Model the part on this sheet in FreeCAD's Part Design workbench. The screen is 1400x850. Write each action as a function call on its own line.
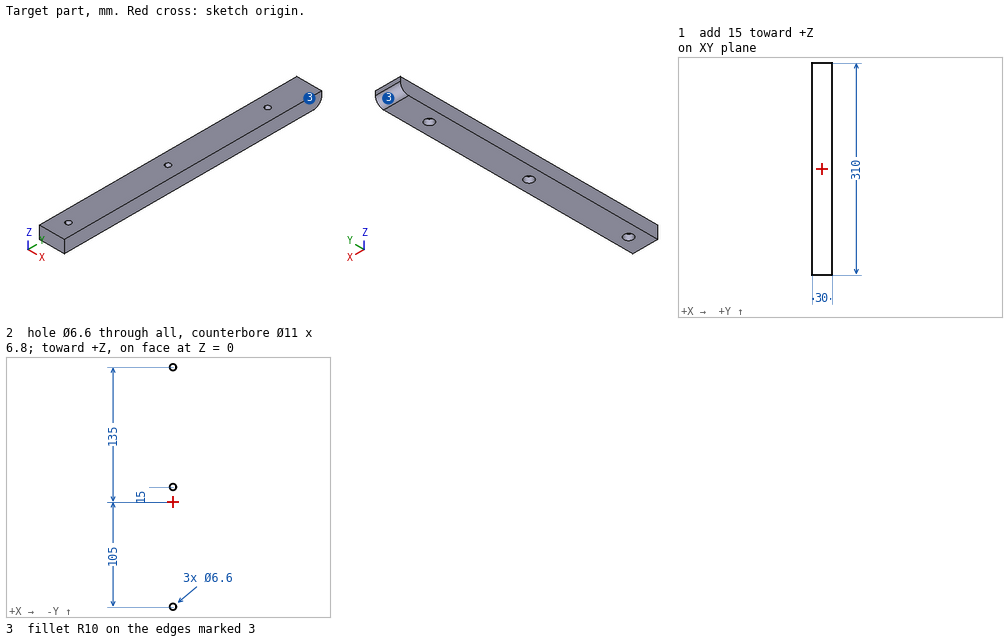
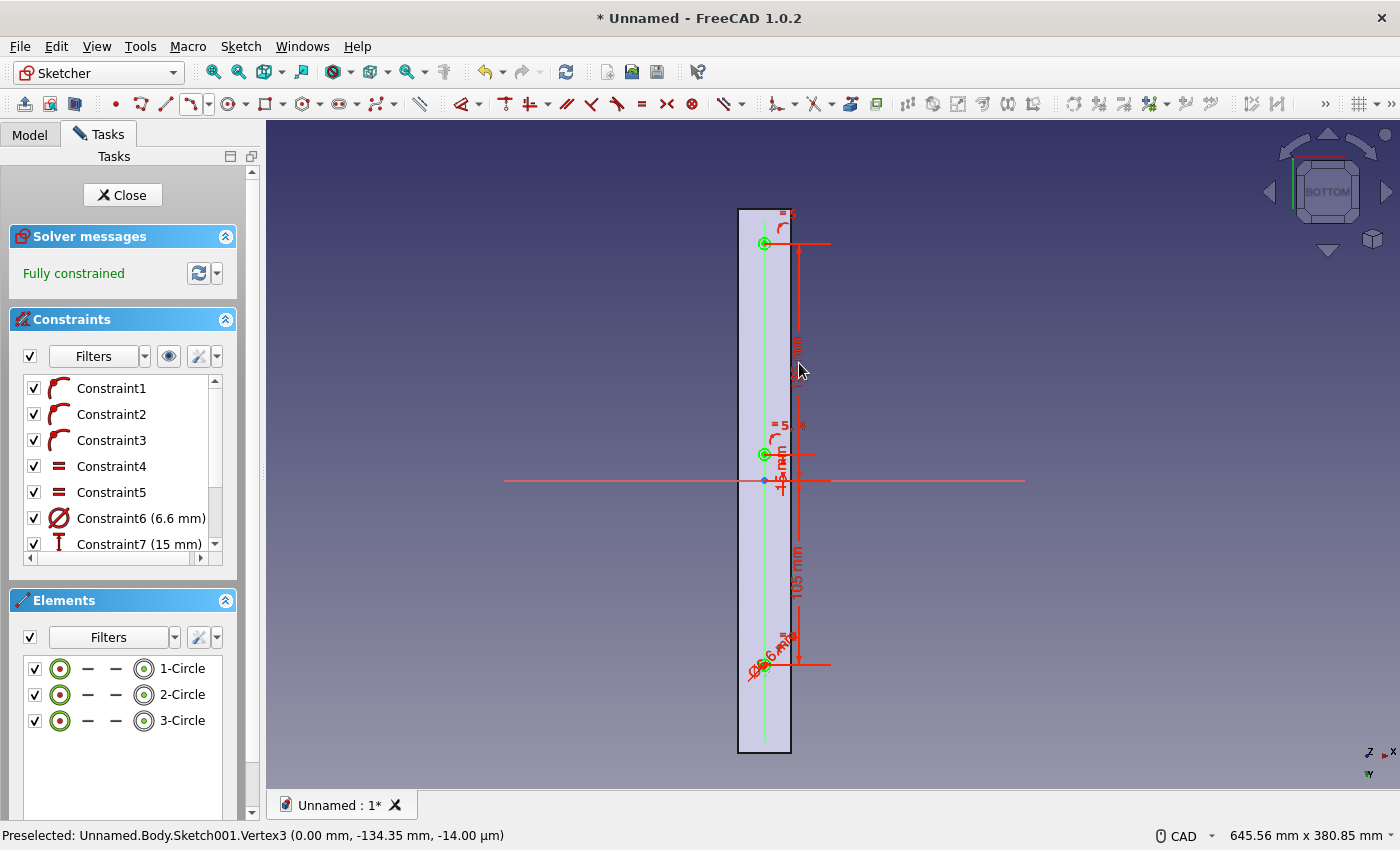
click(123, 195)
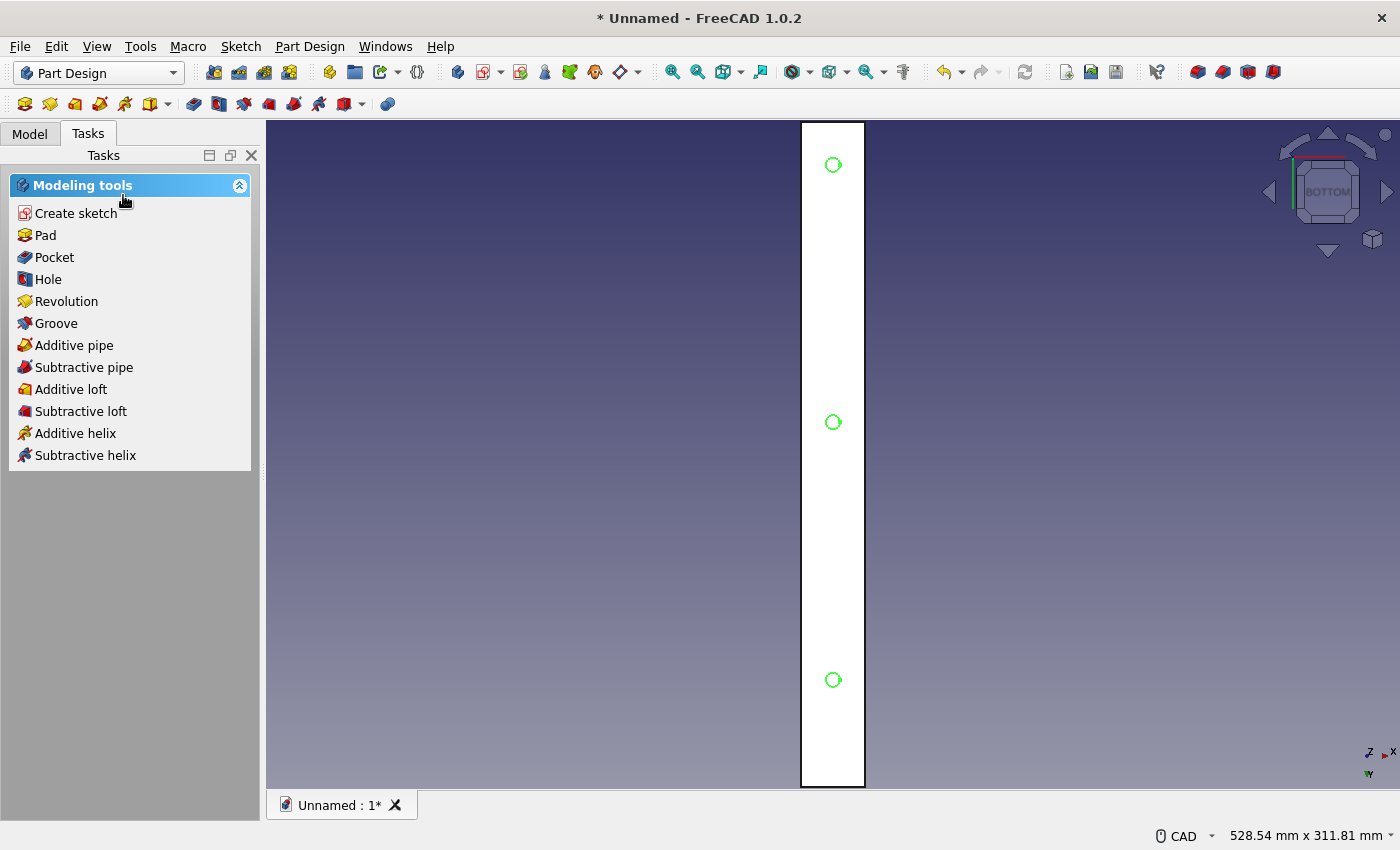
click(219, 104)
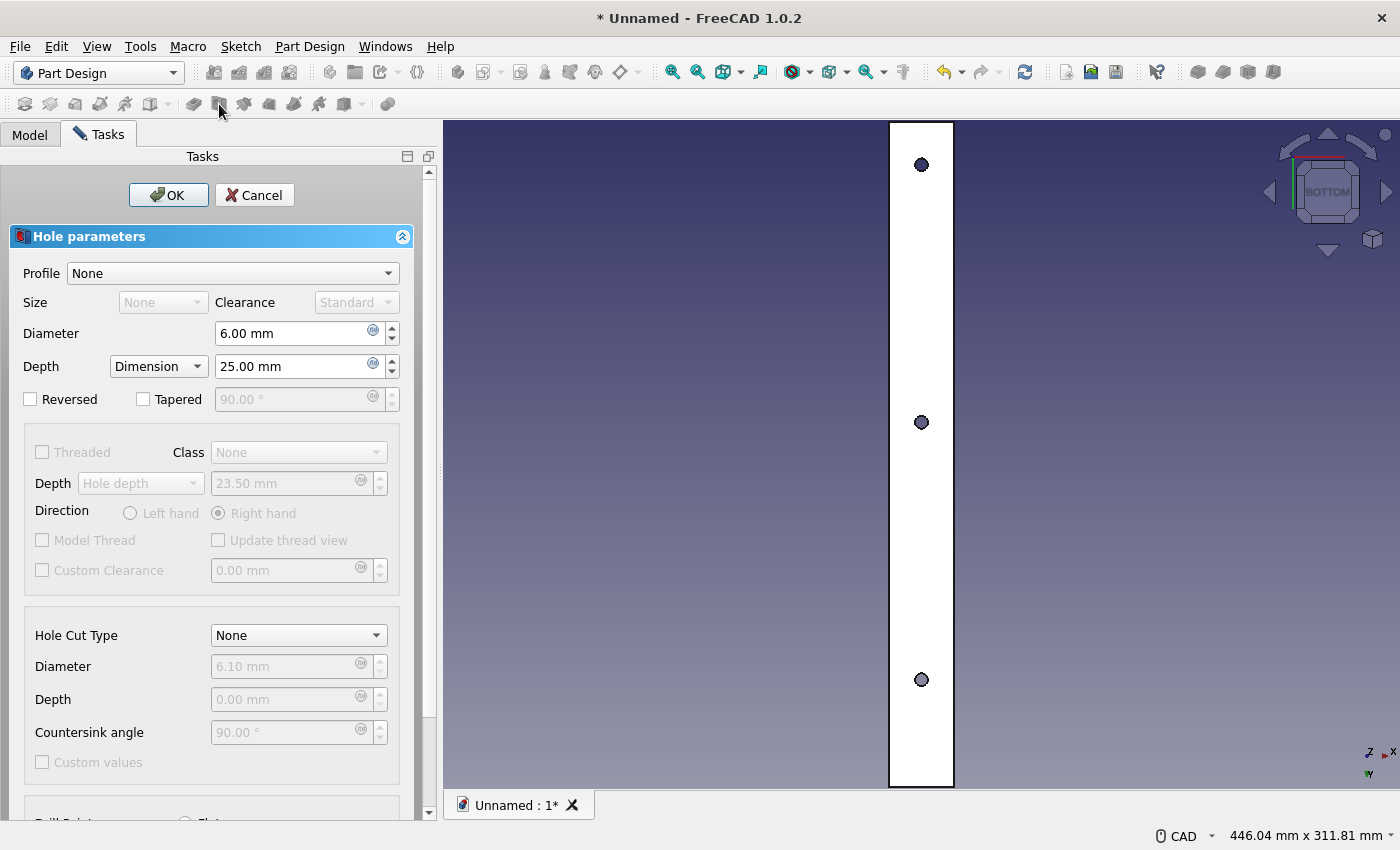
triple_click(300, 334)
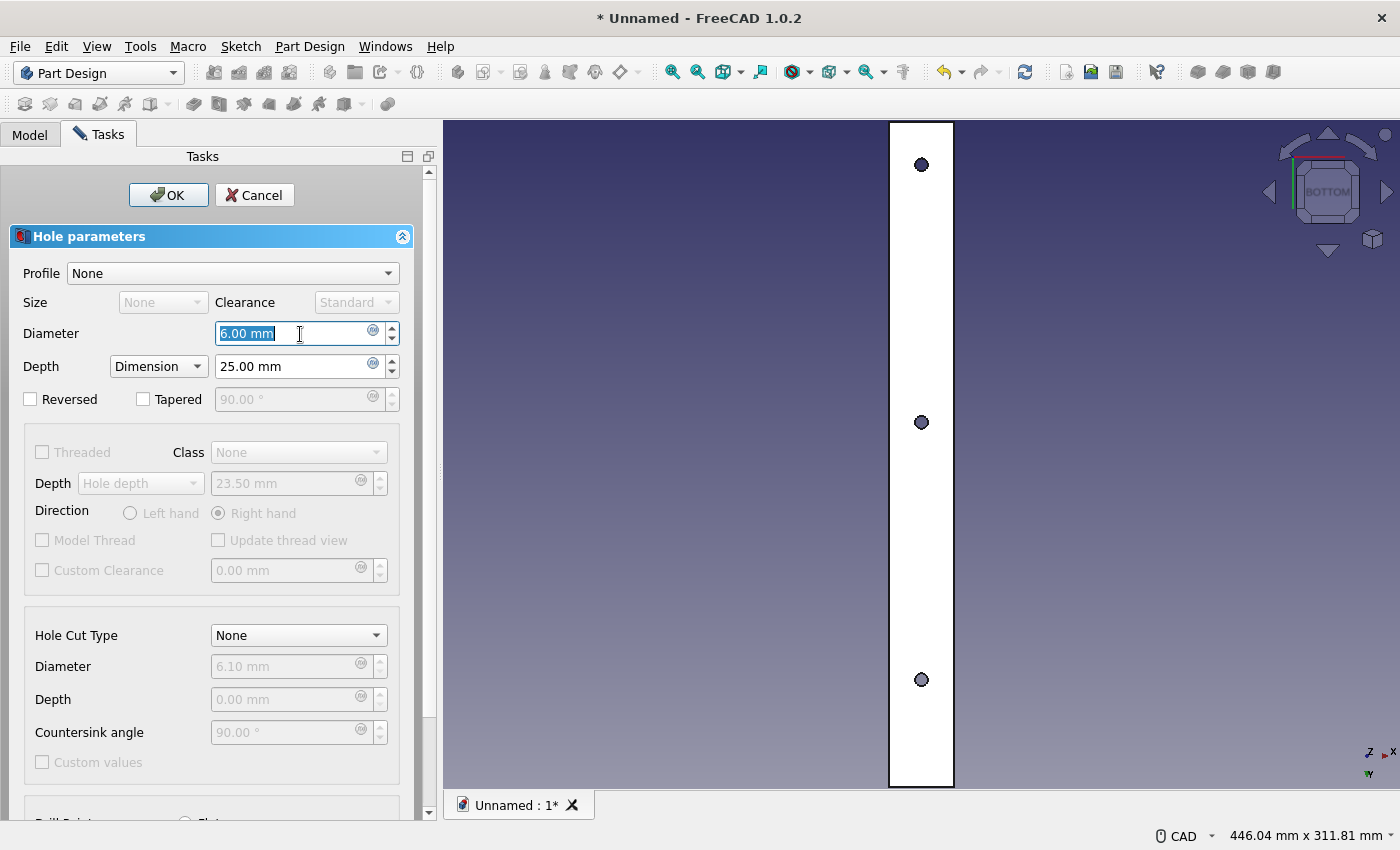
text(6.6)
key(Tab)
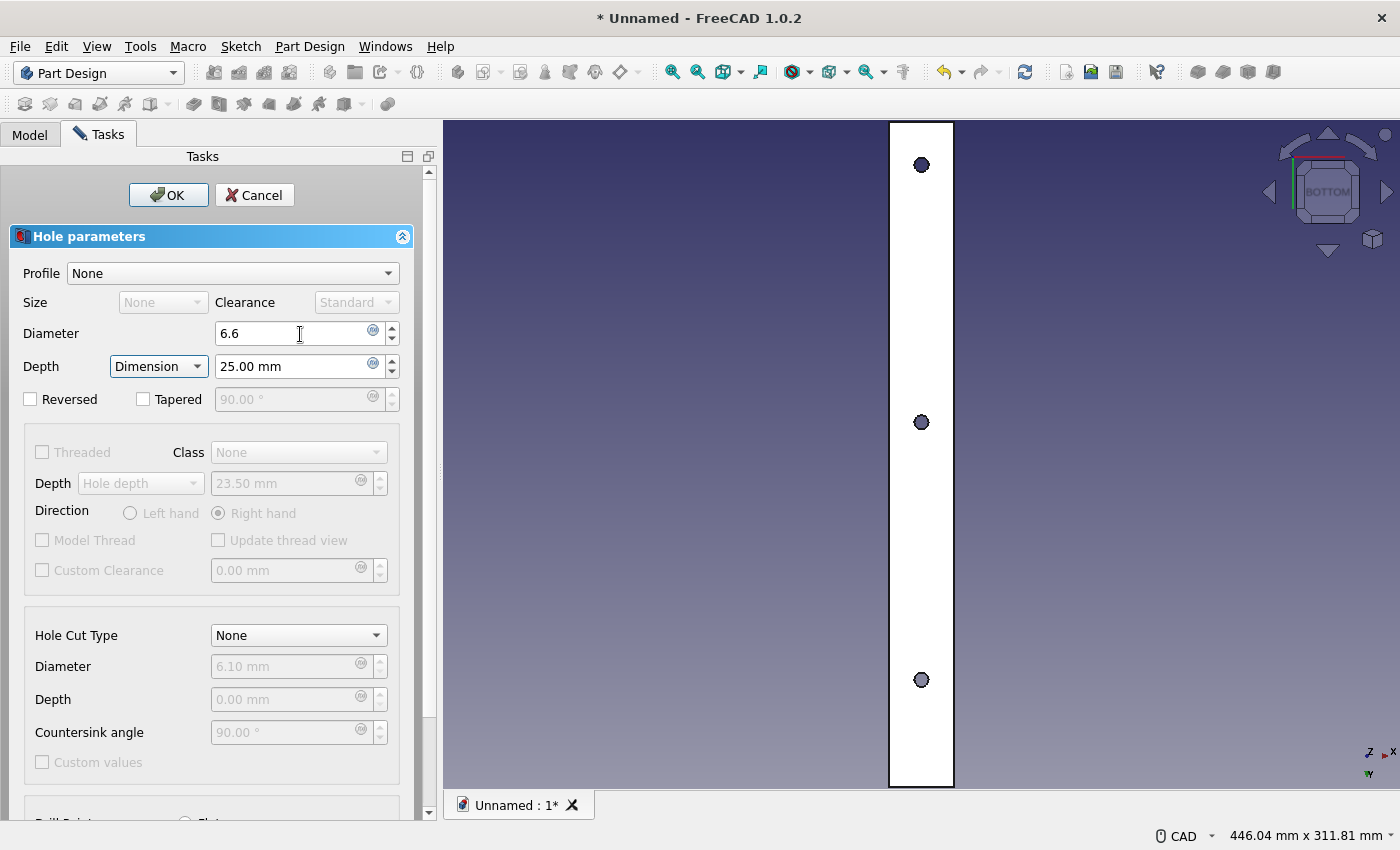
click(160, 366)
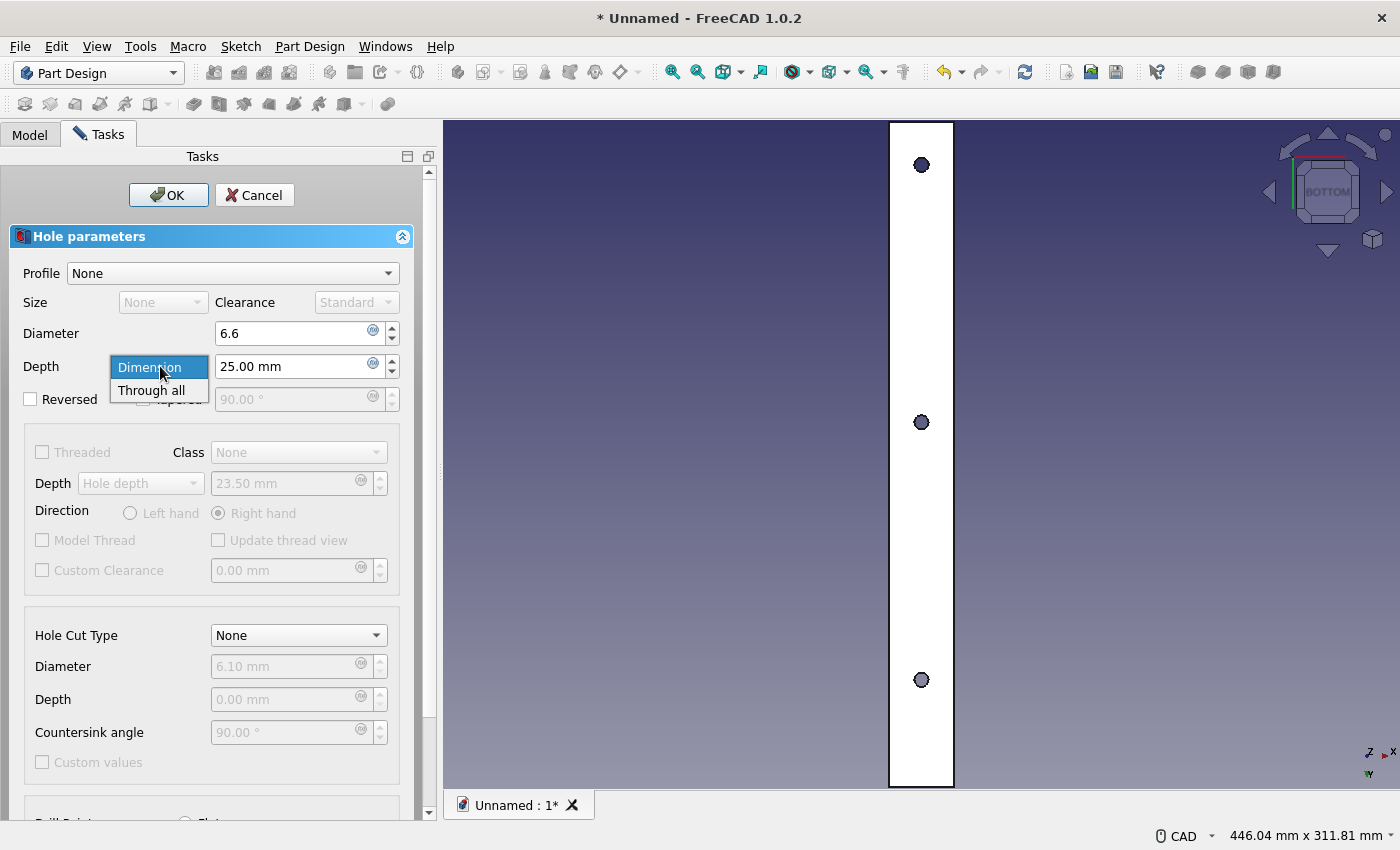
click(158, 390)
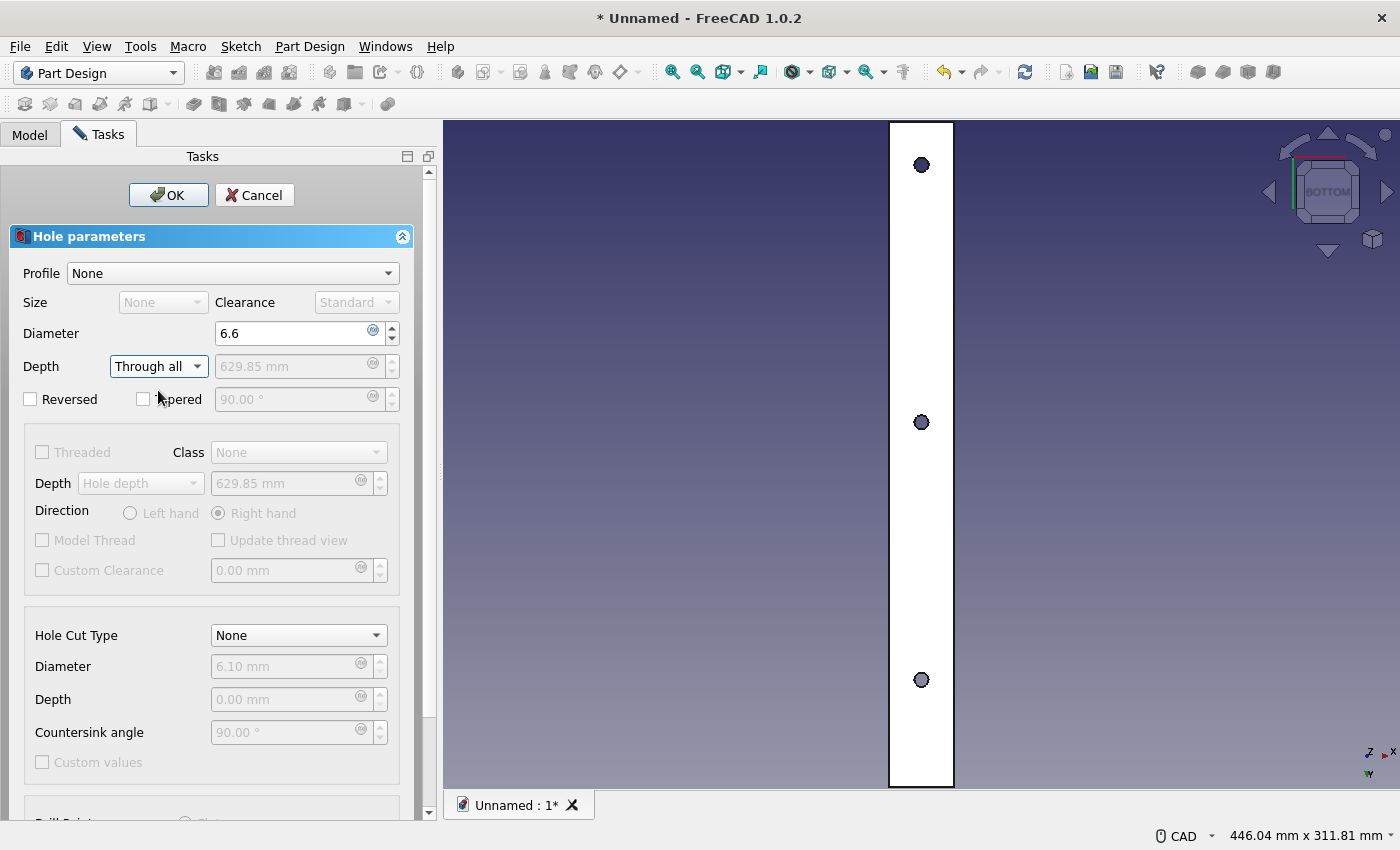
click(300, 636)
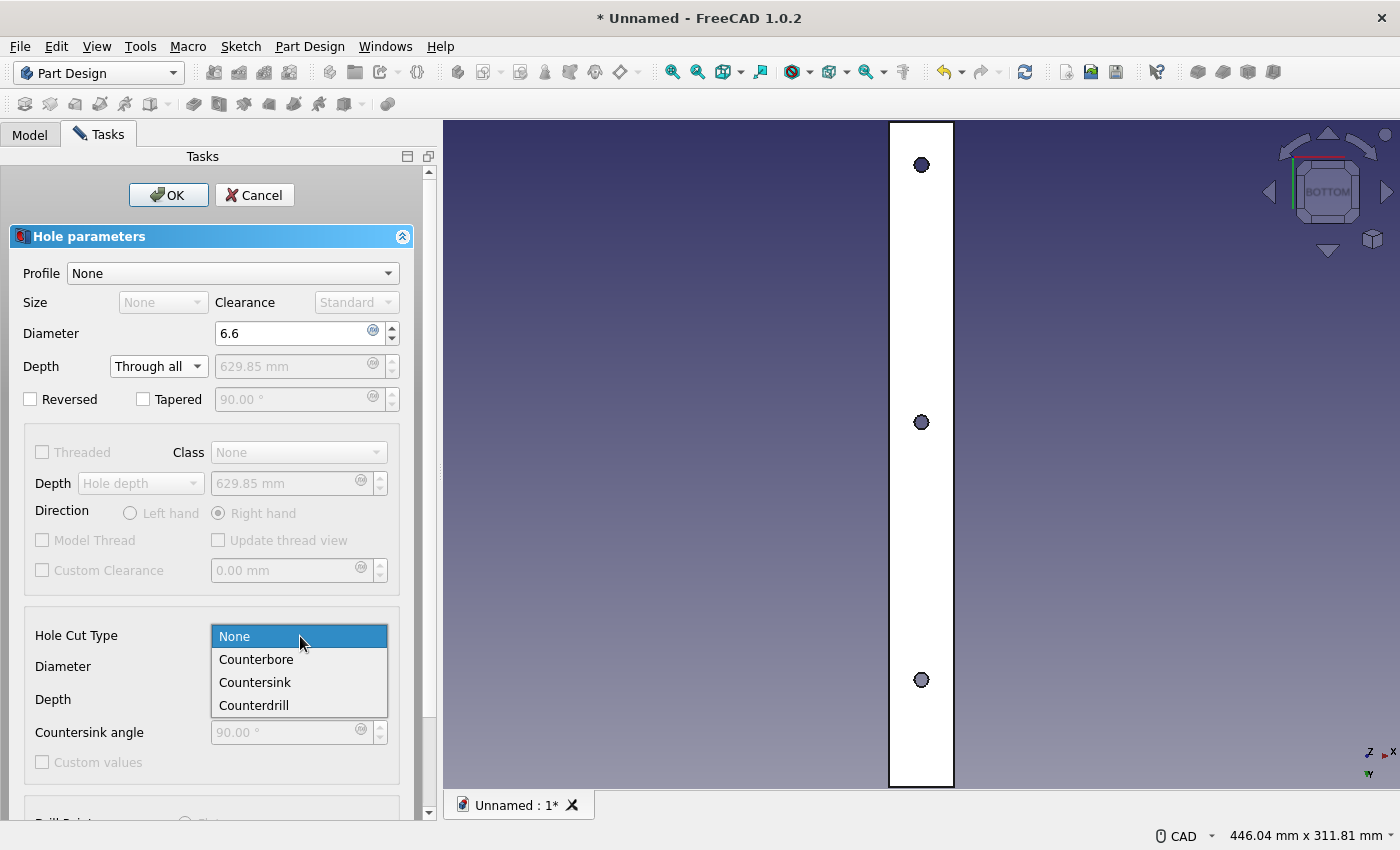
click(298, 660)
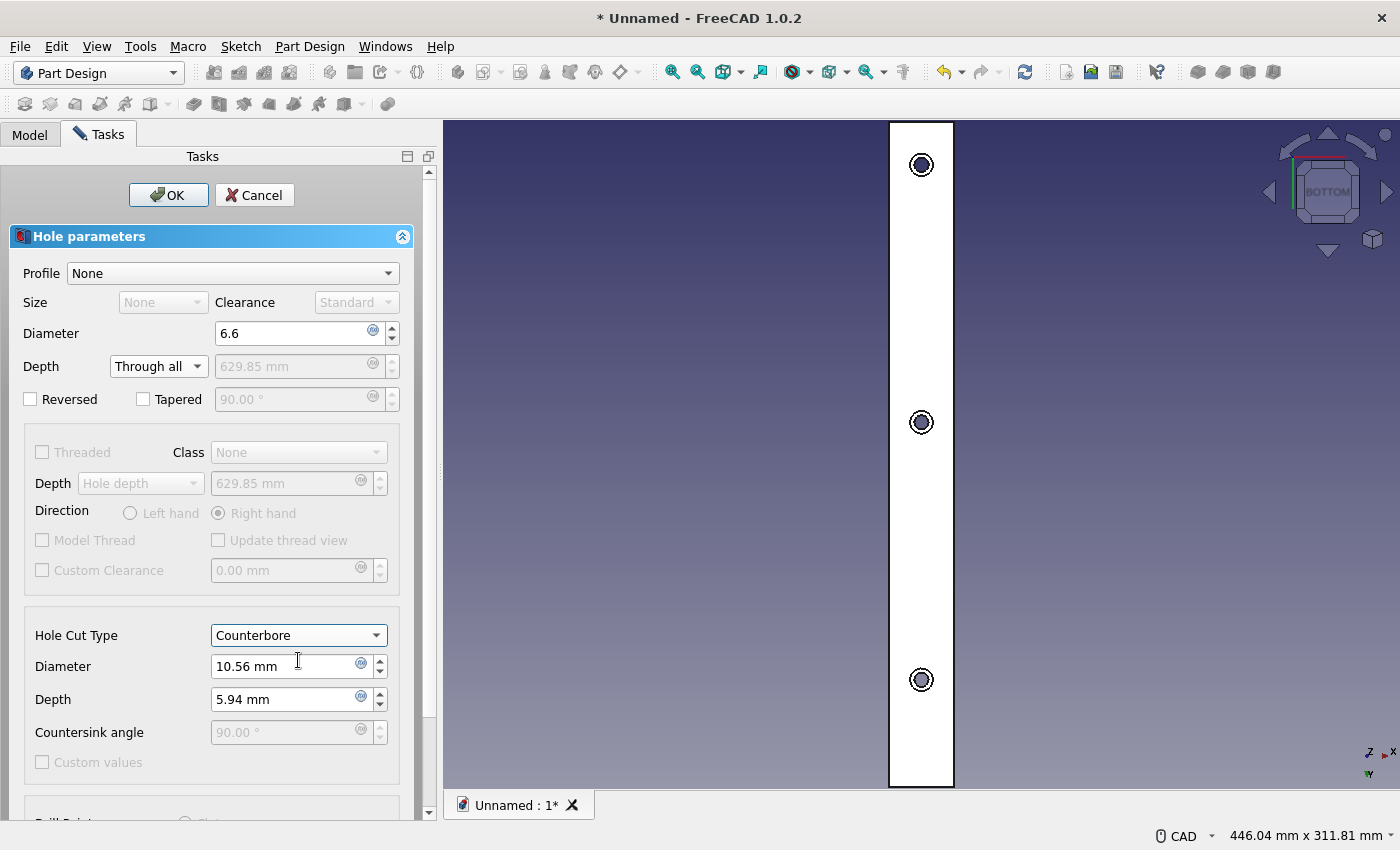
triple_click(292, 666)